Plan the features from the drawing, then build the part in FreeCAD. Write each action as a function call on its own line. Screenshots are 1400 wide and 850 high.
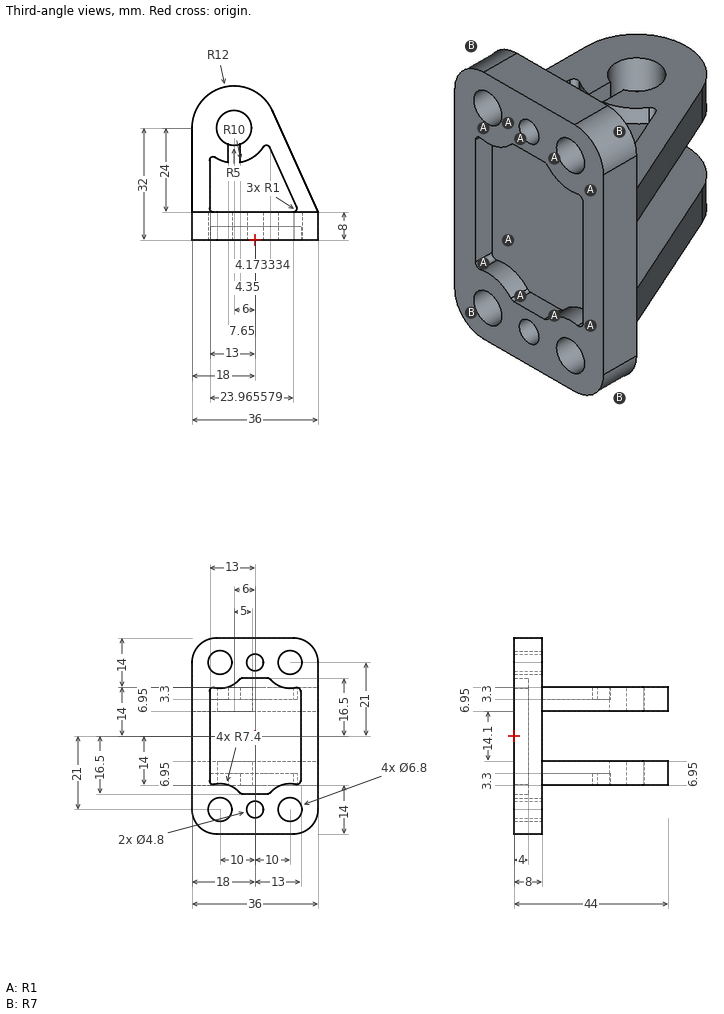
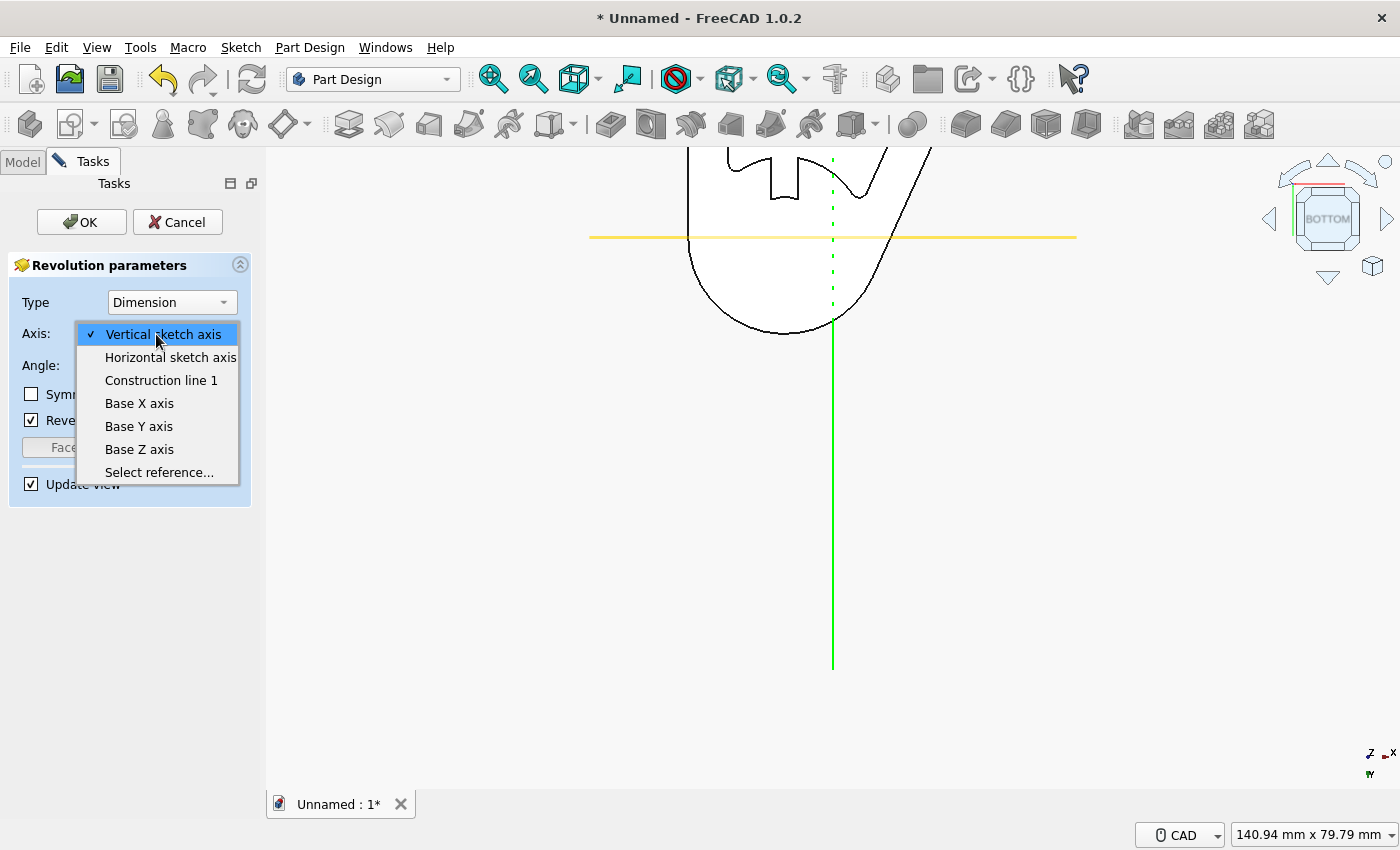
click(156, 380)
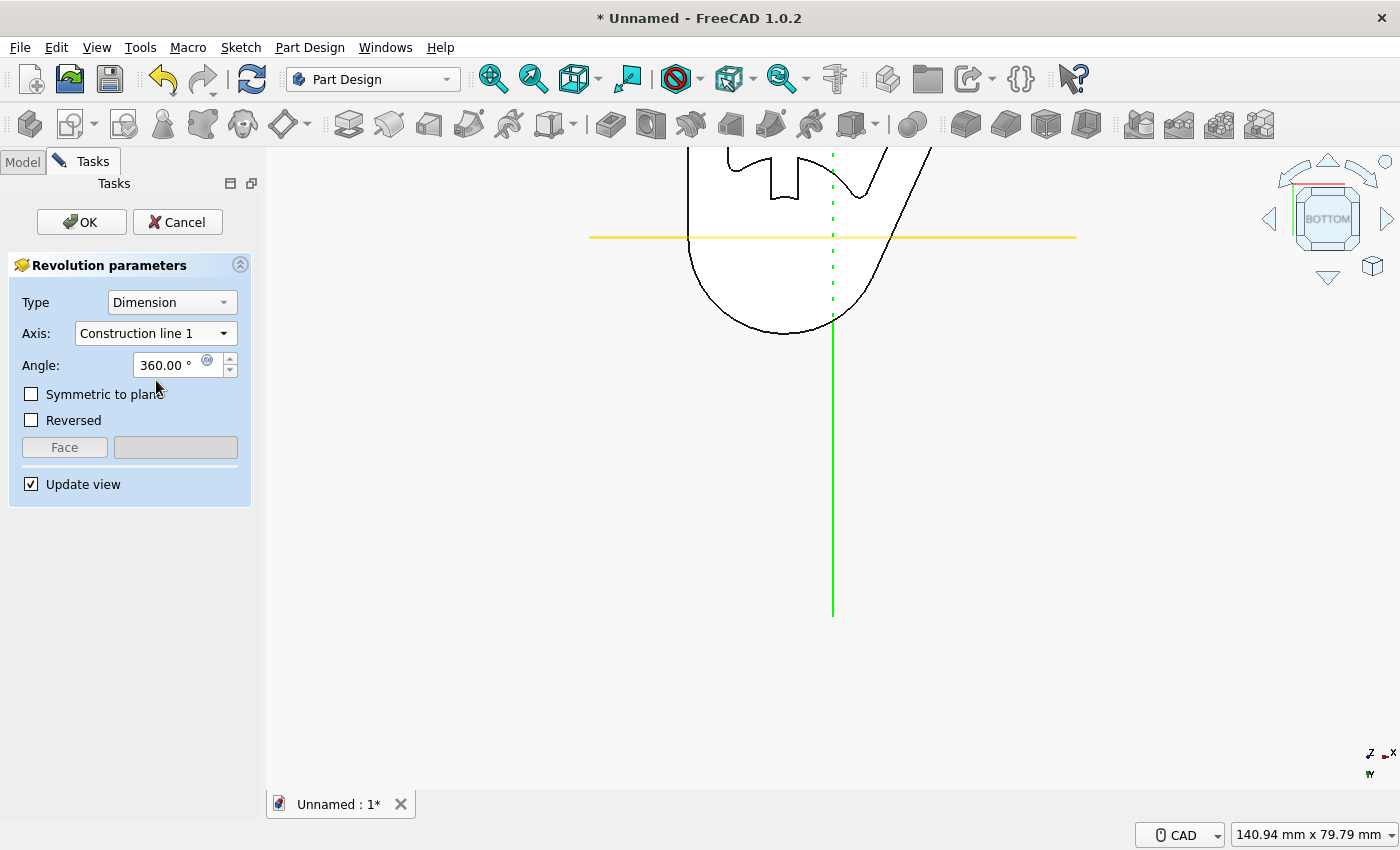
click(82, 222)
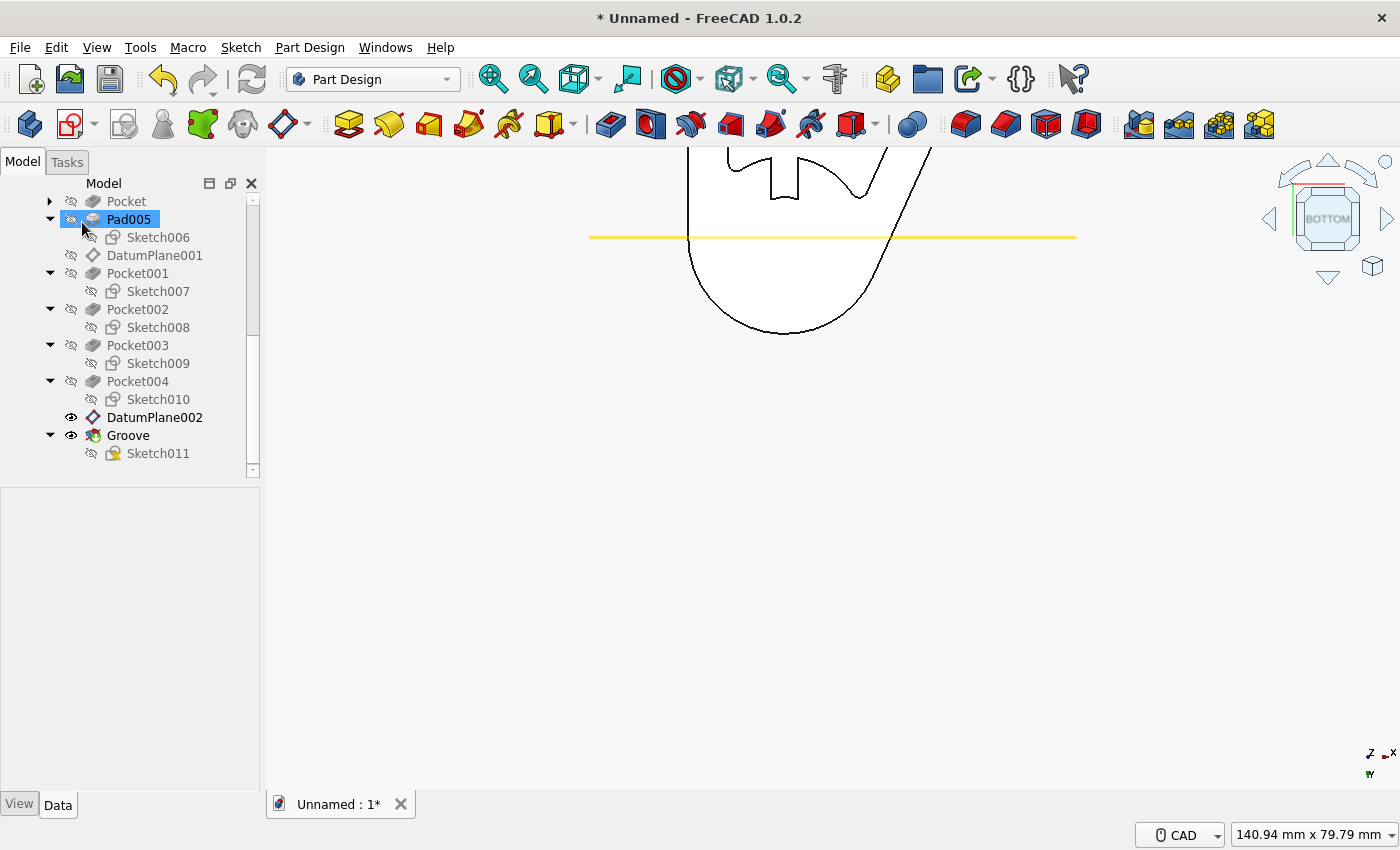
click(116, 417)
key(space)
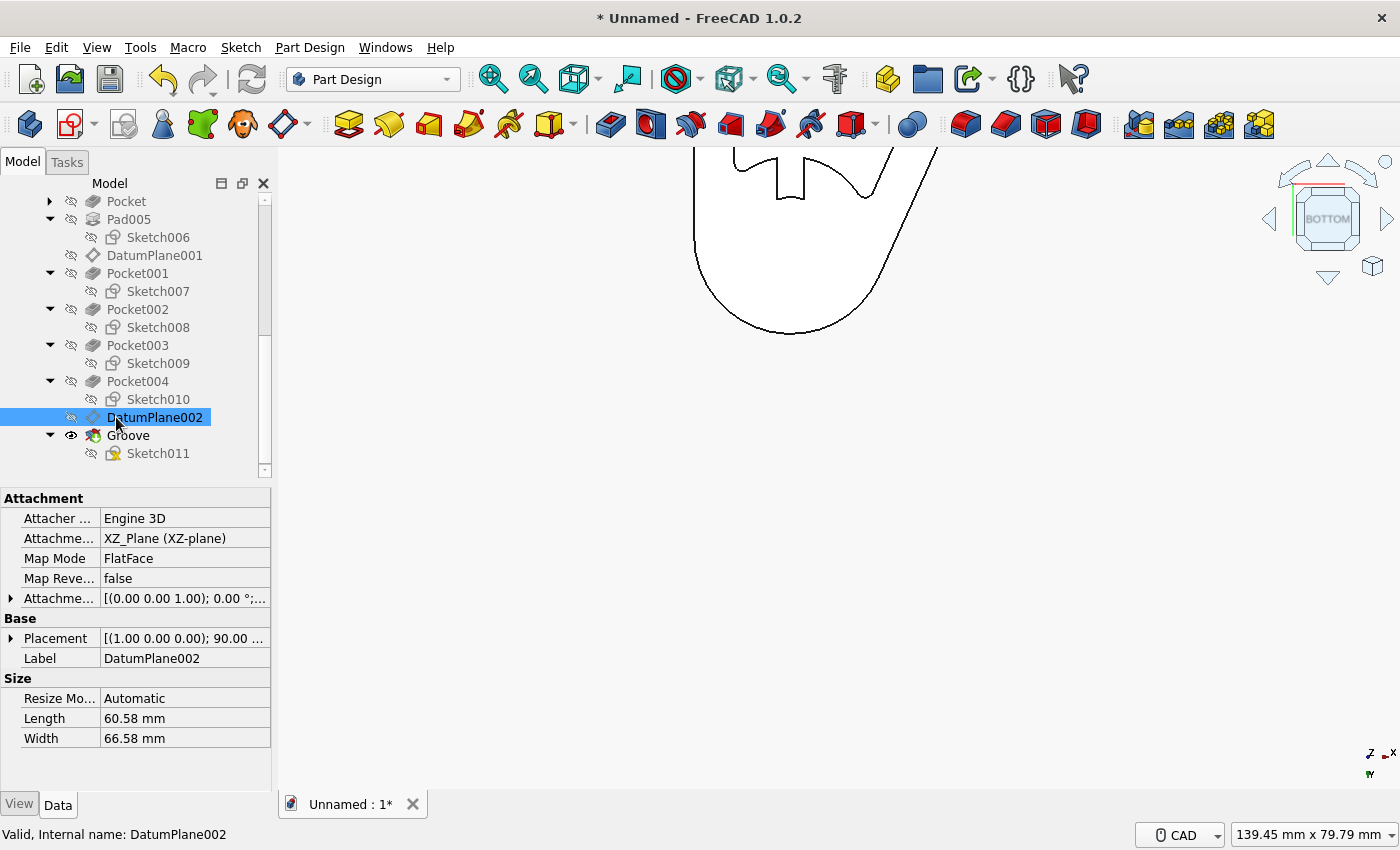
key(v)
key(f)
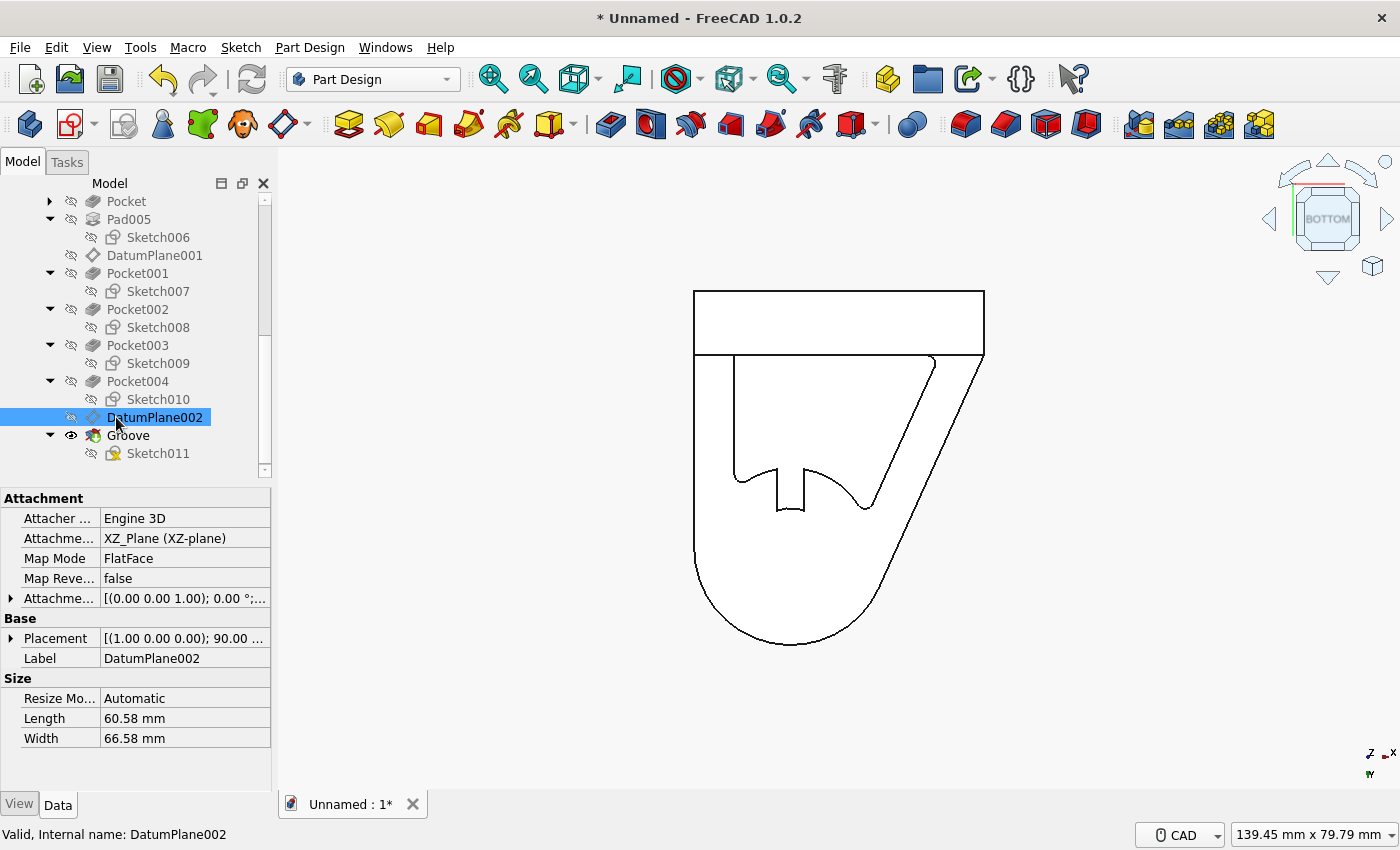
scroll(140, 323, down, 3)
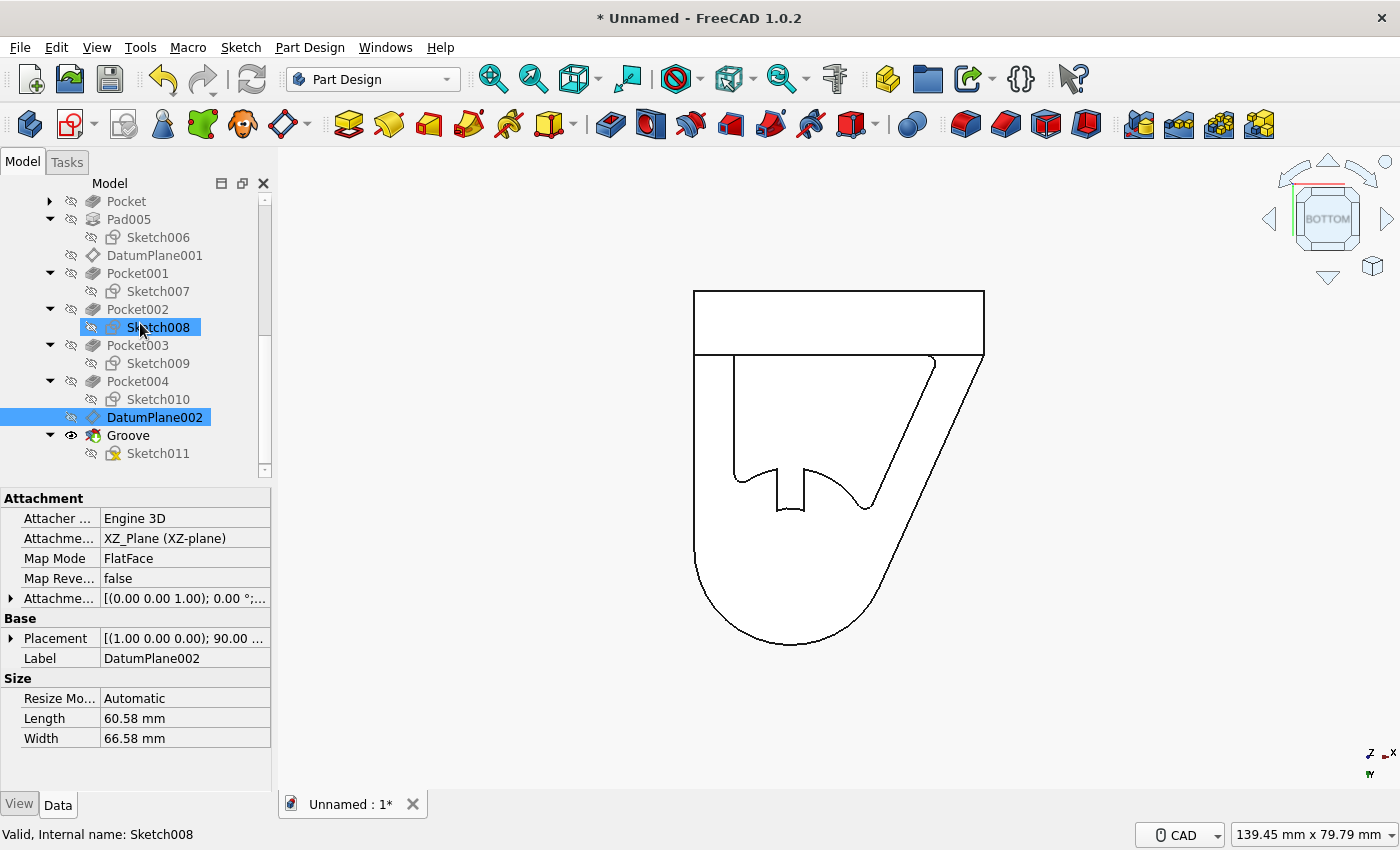
scroll(140, 323, up, 15)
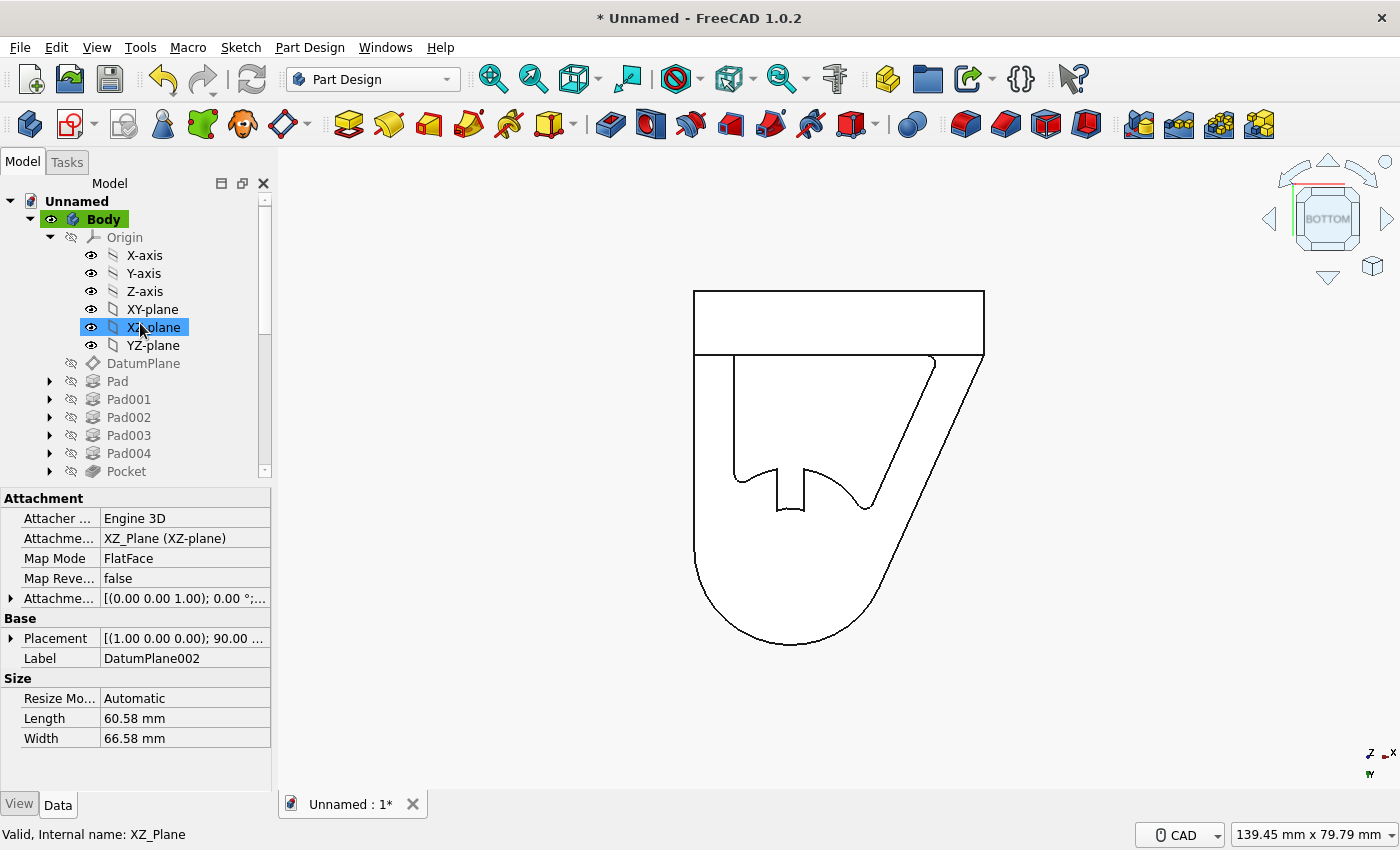
click(136, 327)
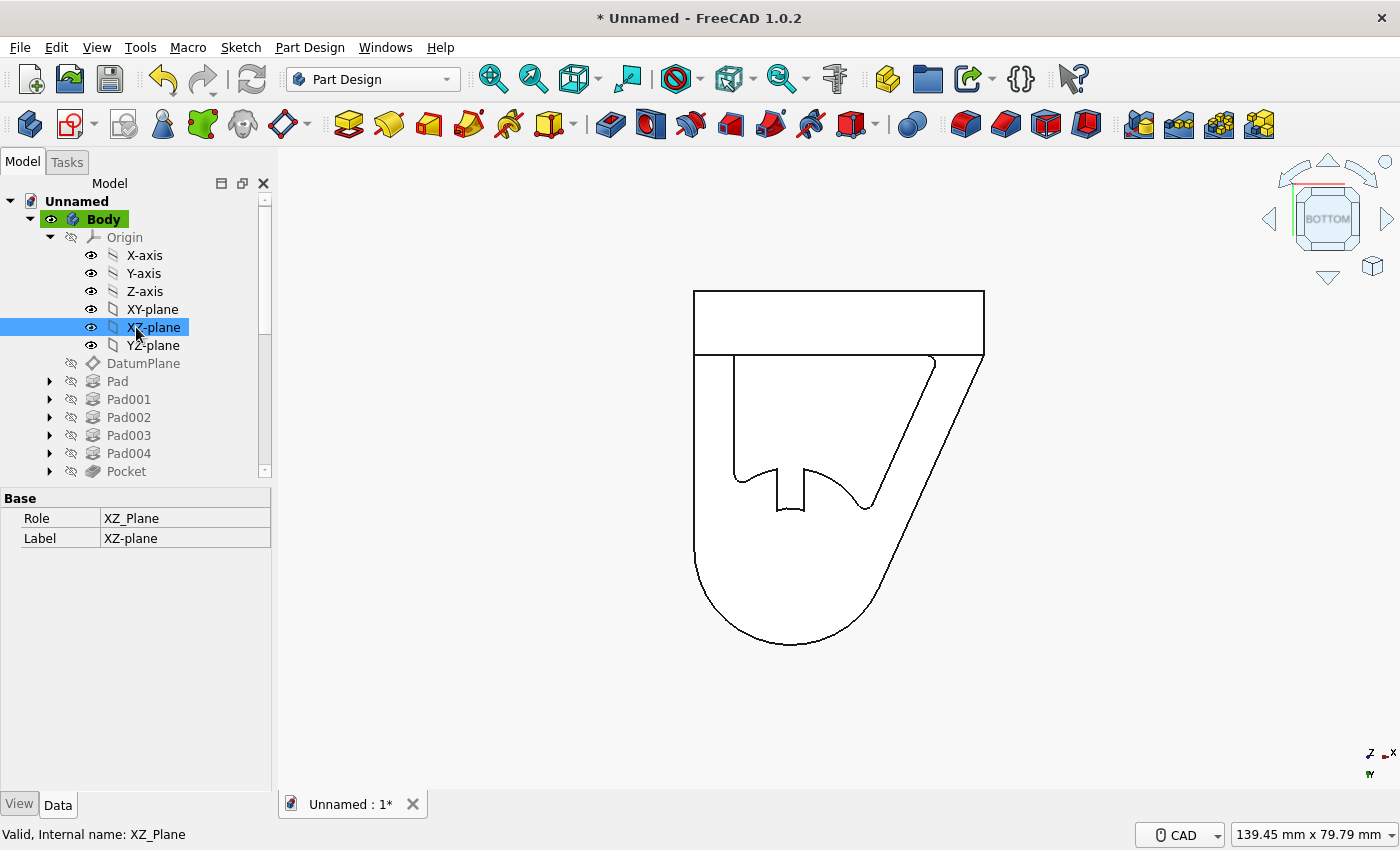
click(284, 124)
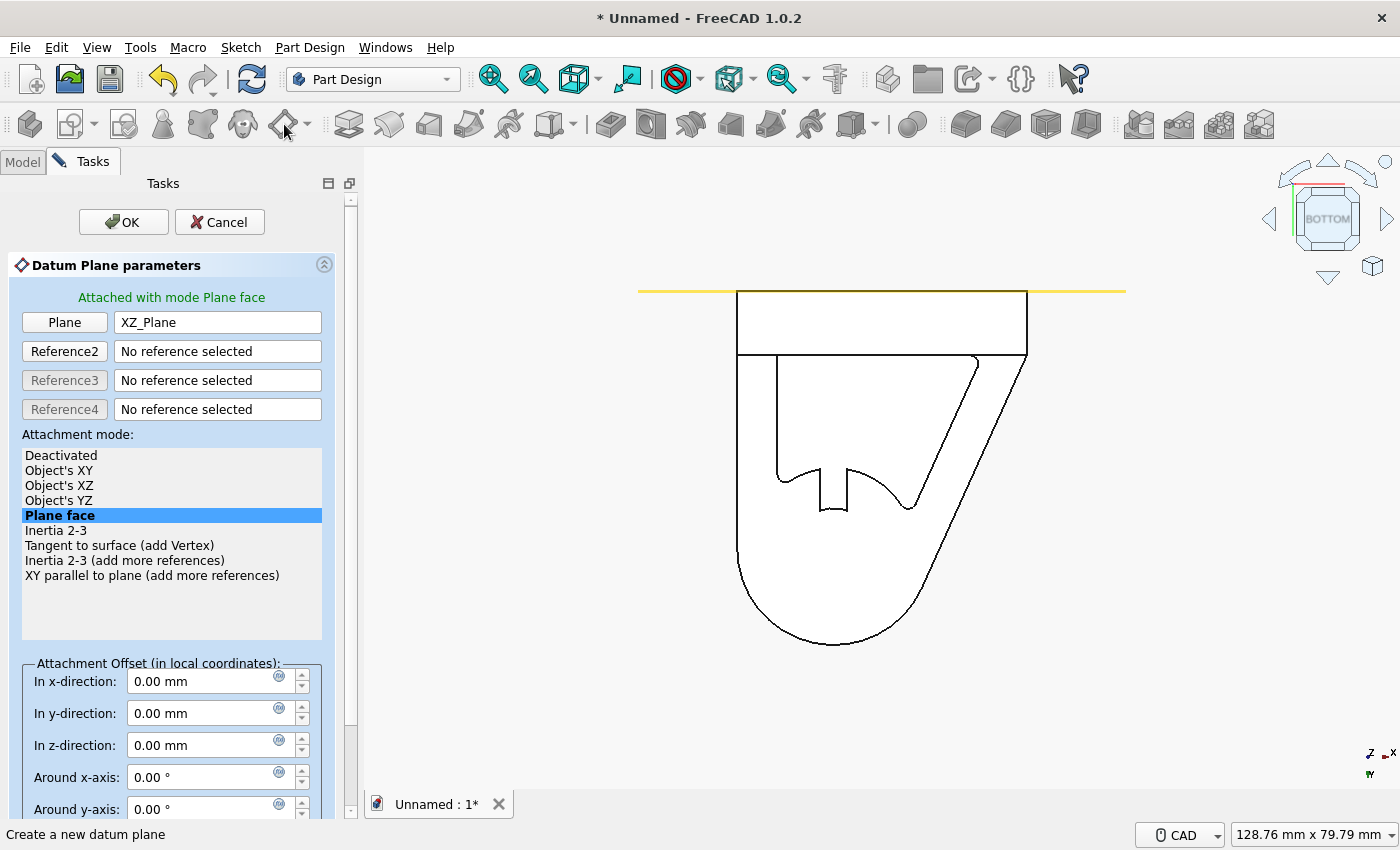
triple_click(210, 745)